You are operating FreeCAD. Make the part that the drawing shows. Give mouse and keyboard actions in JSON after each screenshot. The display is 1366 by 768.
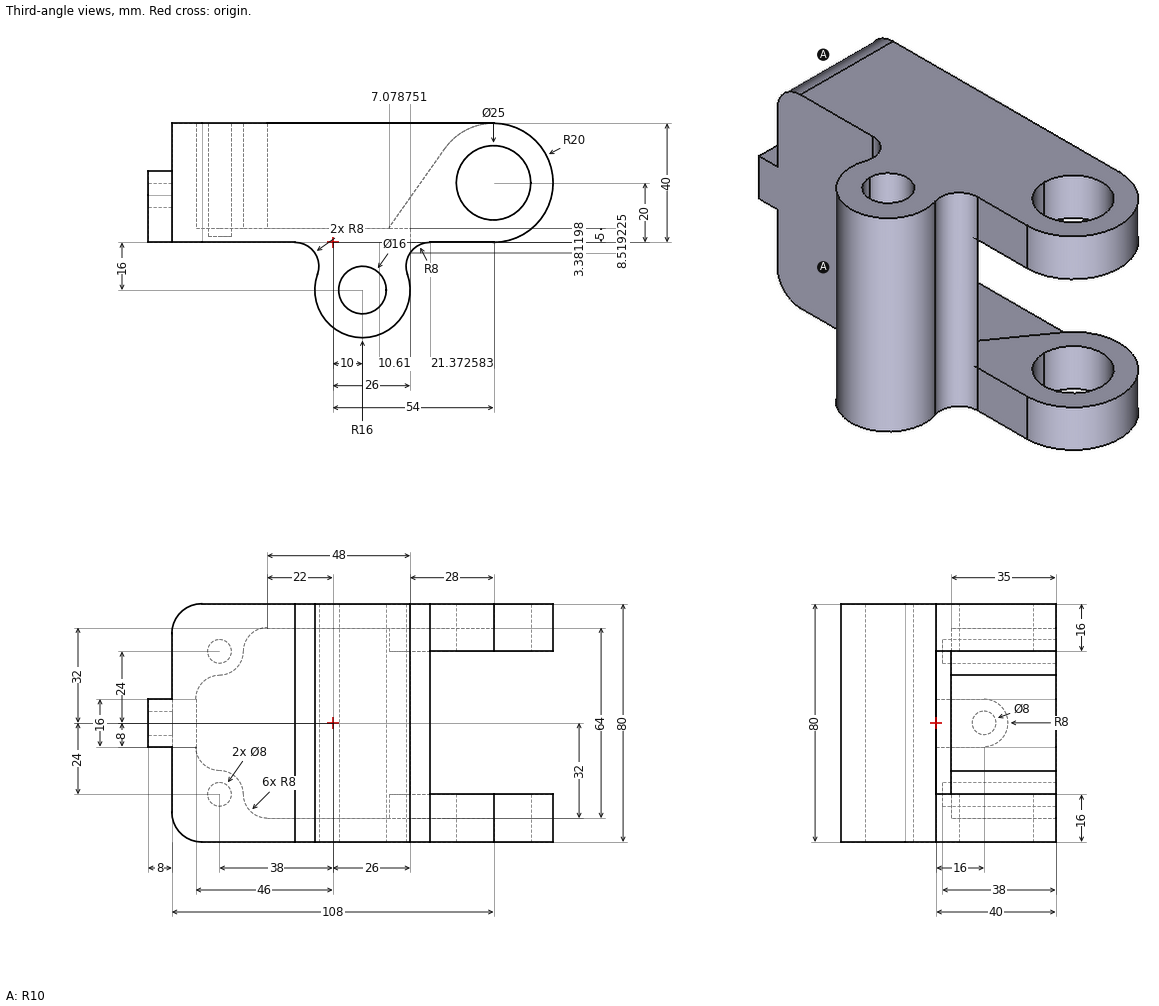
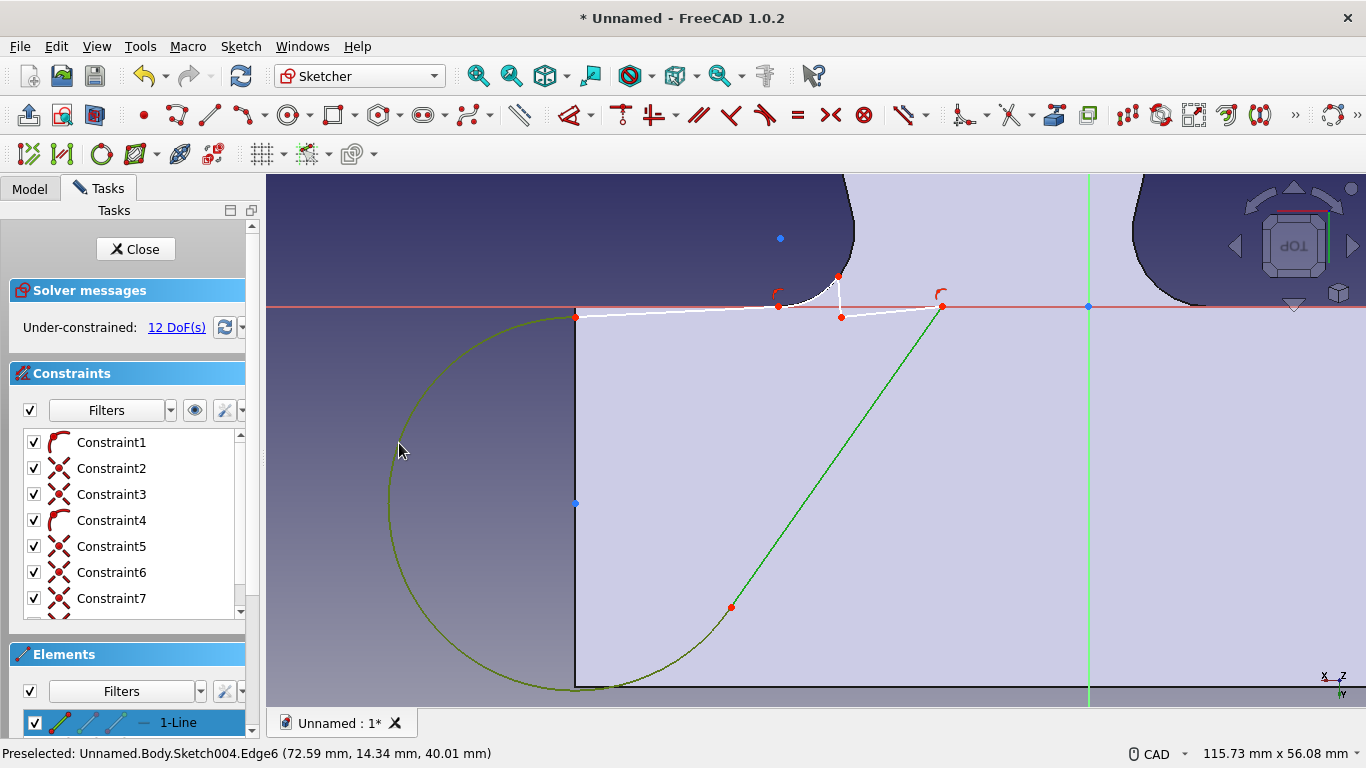
{"action": "key", "text": "t"}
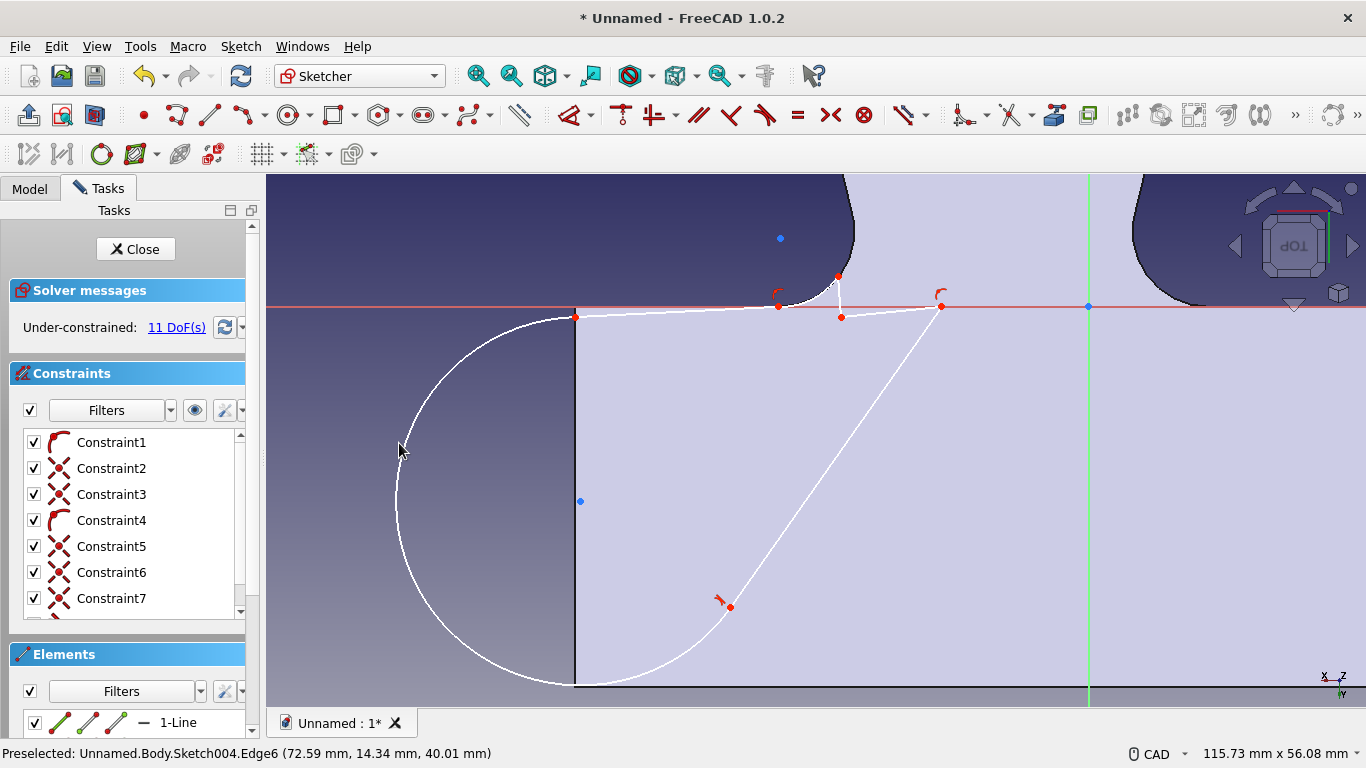
{"action": "left_click", "coordinate": [717, 310]}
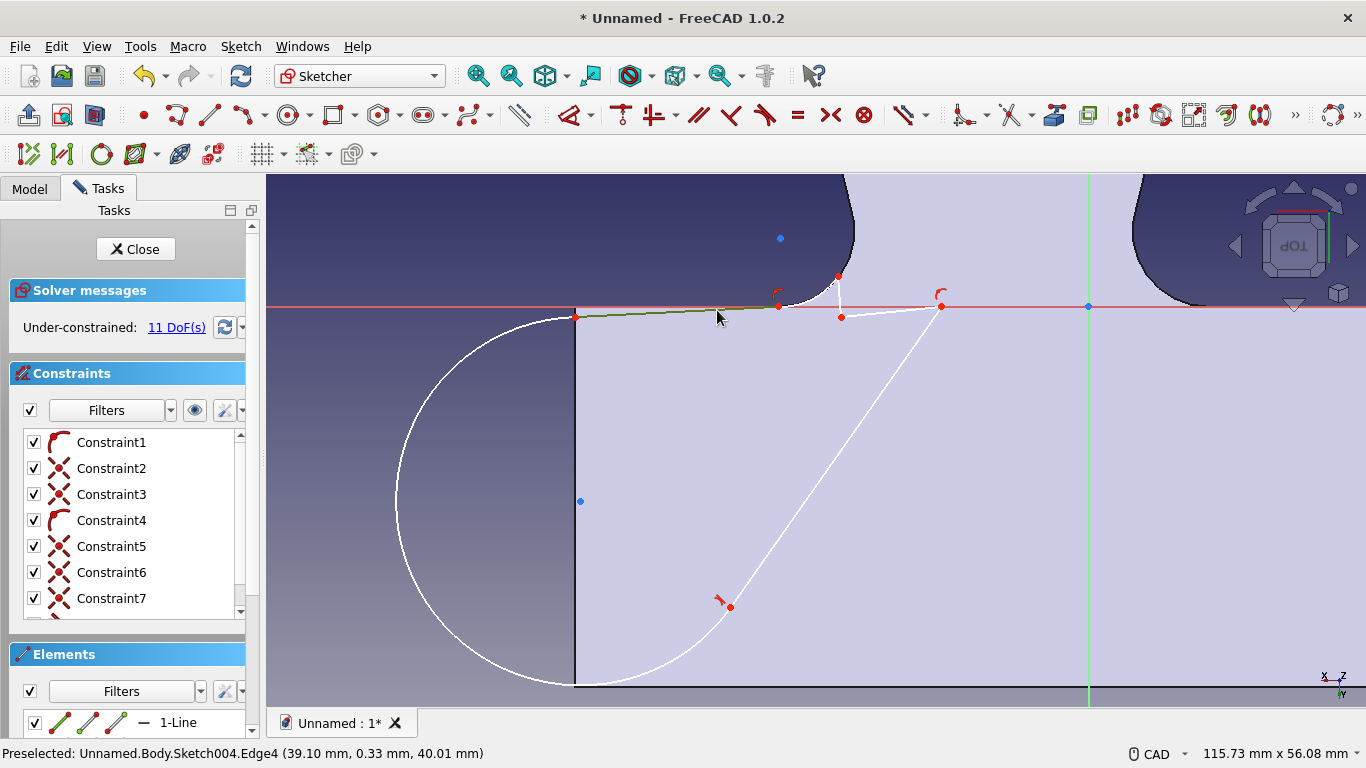
{"action": "left_click", "coordinate": [799, 304]}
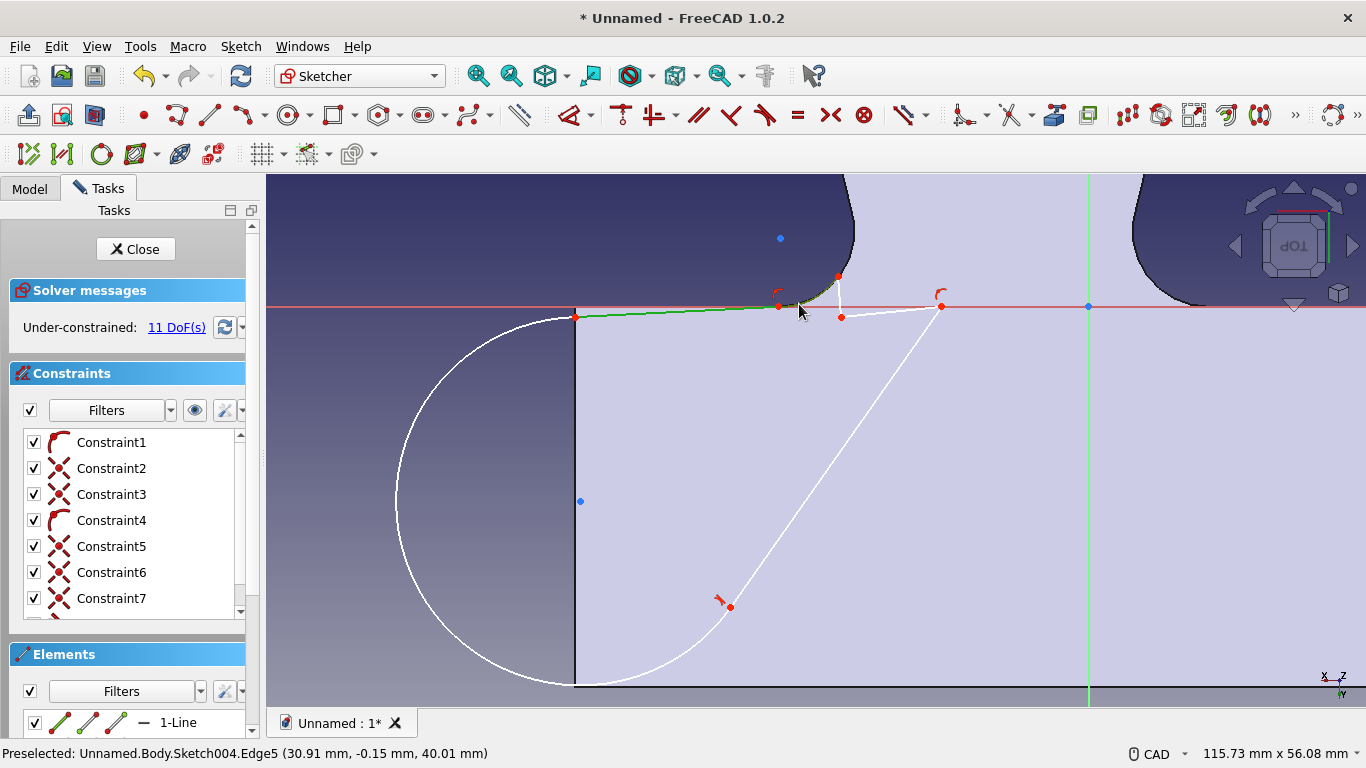
{"action": "key", "text": "t"}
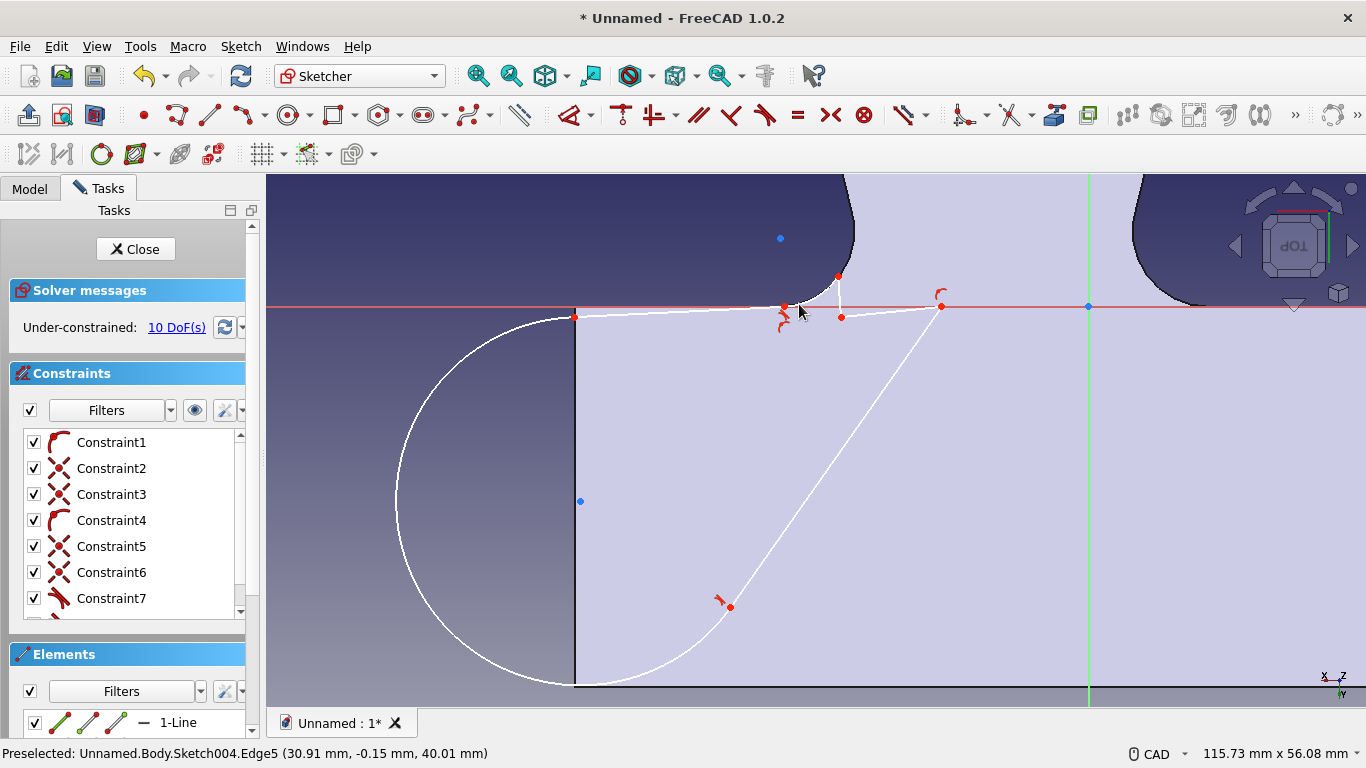
{"action": "left_click", "coordinate": [722, 310]}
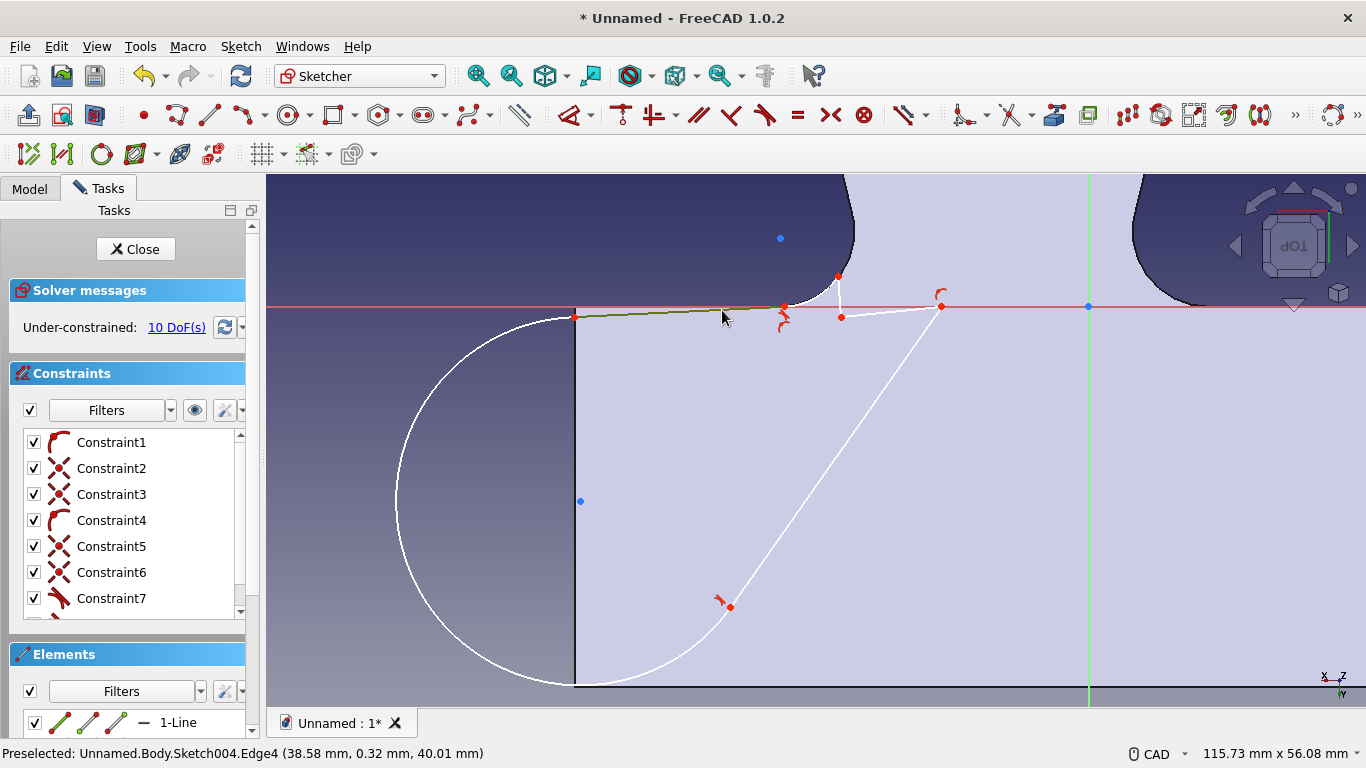
{"action": "left_click", "coordinate": [405, 443]}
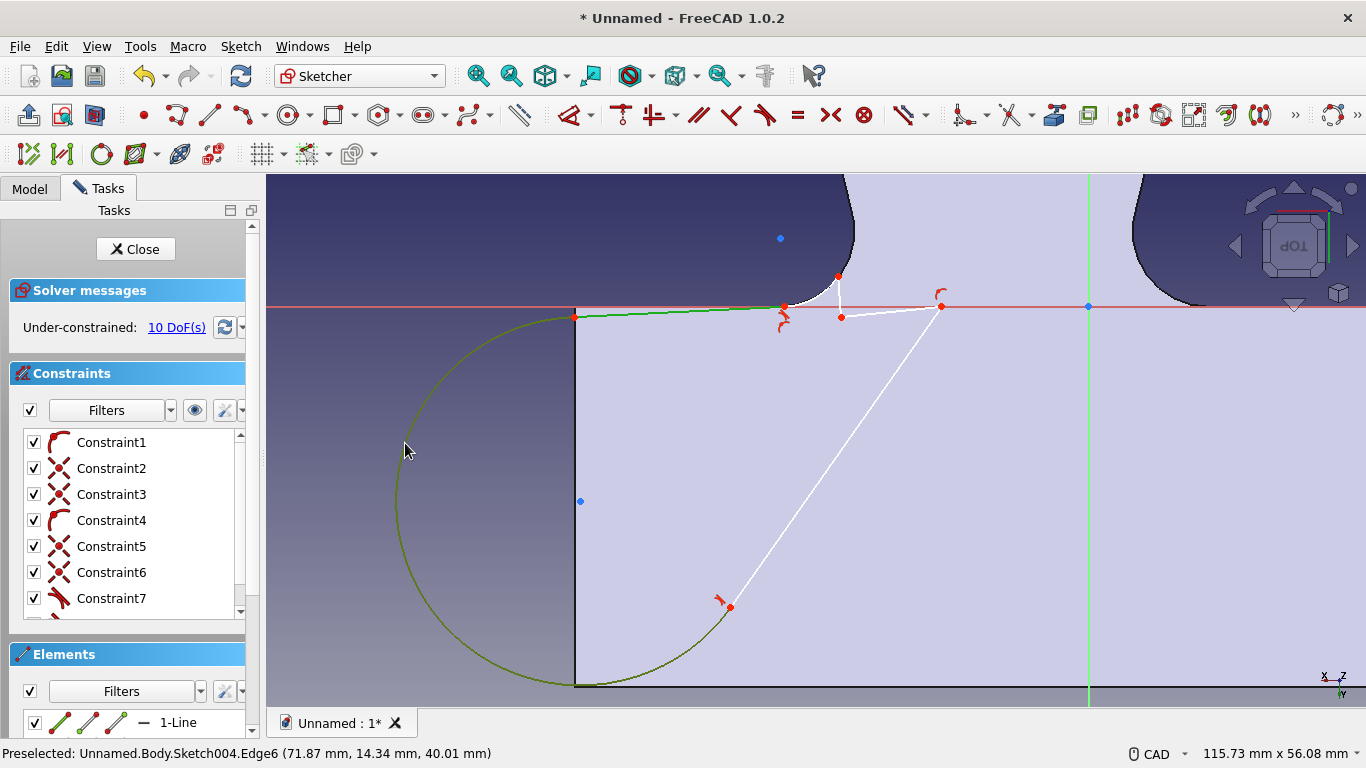
{"action": "key", "text": "t"}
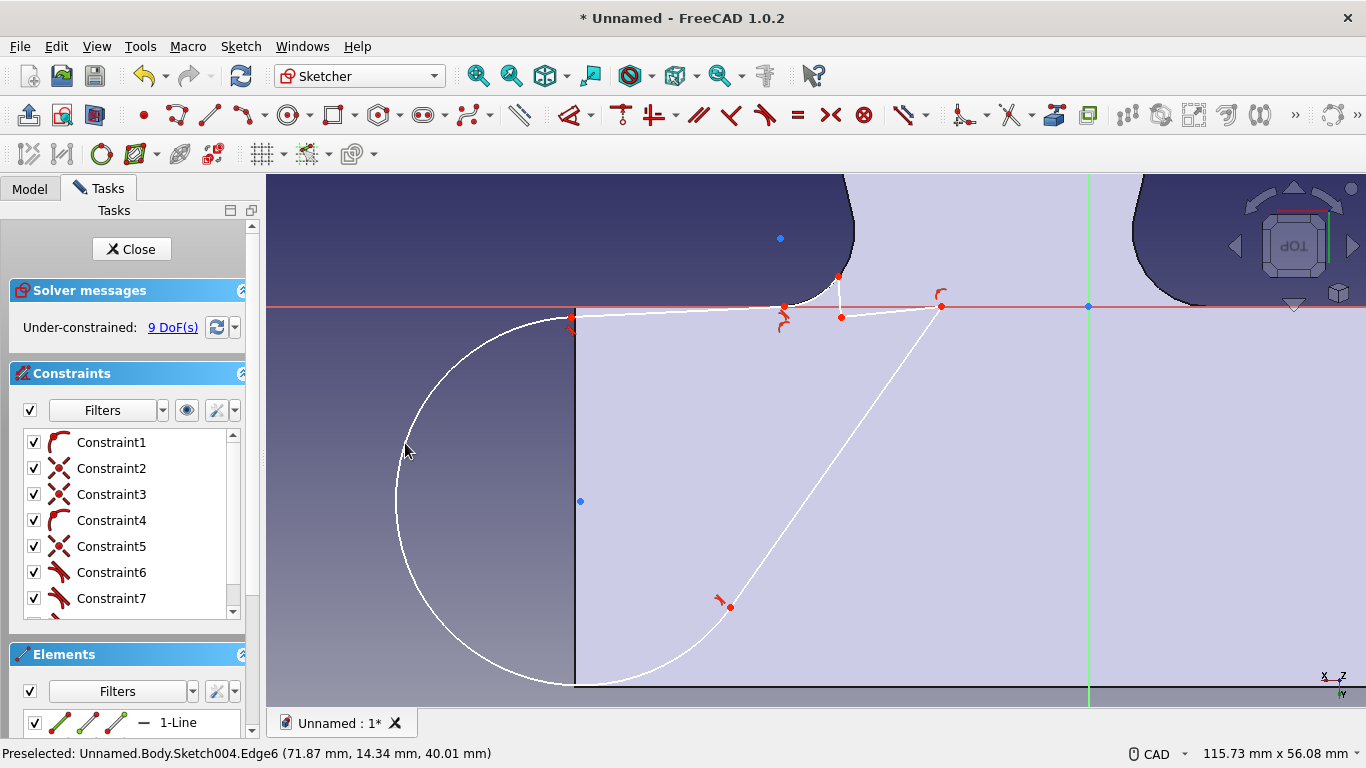
{"action": "left_click", "coordinate": [912, 310]}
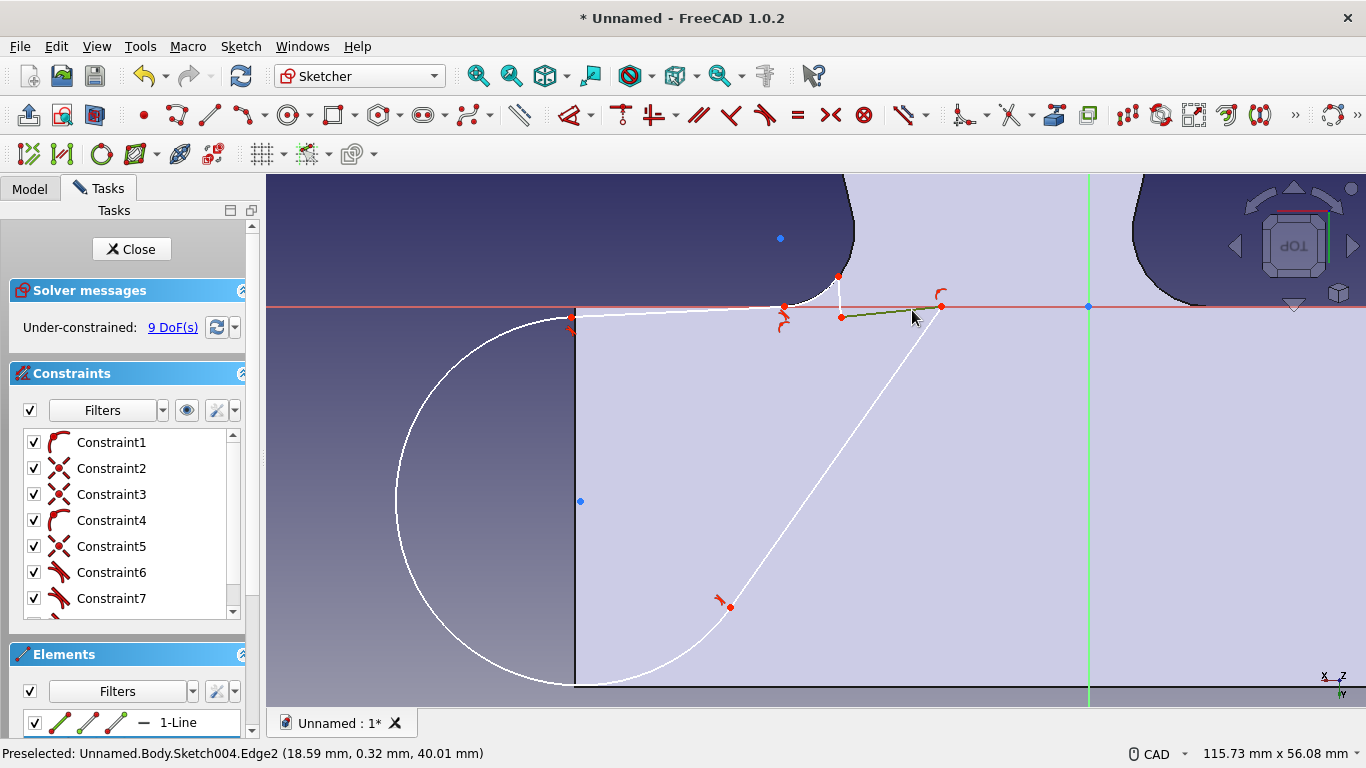
{"action": "key", "text": "h"}